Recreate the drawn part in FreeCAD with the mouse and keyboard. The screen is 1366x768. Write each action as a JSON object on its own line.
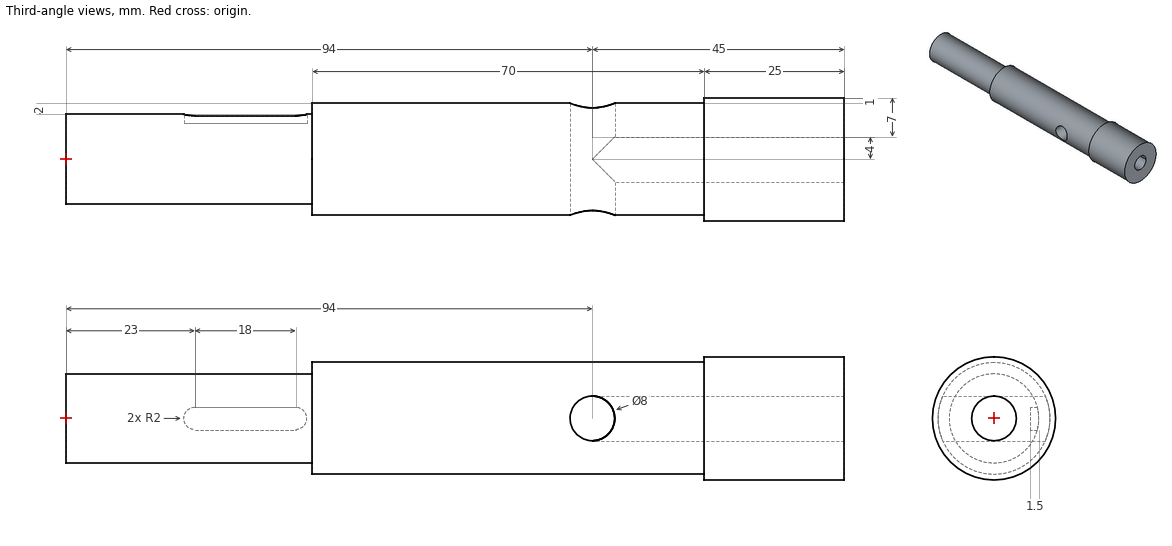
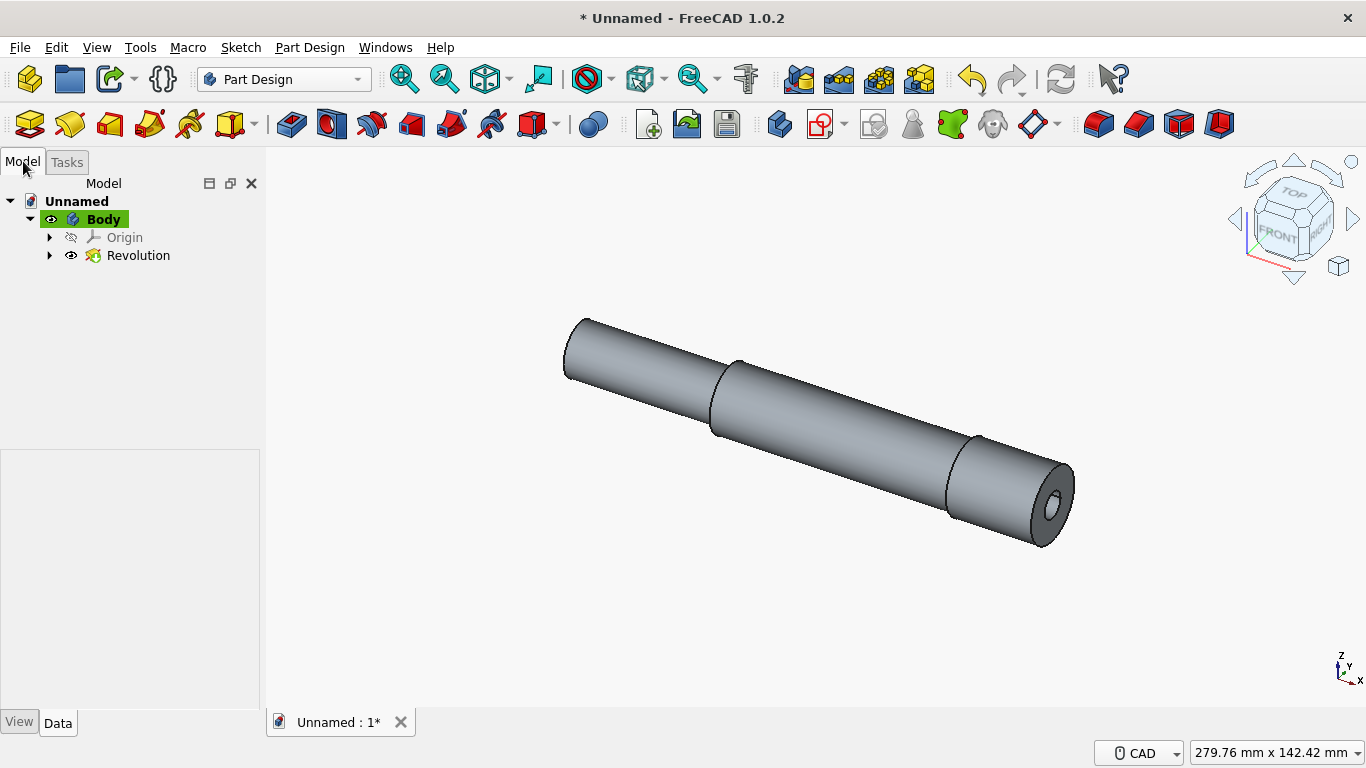
{"action": "left_click", "coordinate": [50, 237]}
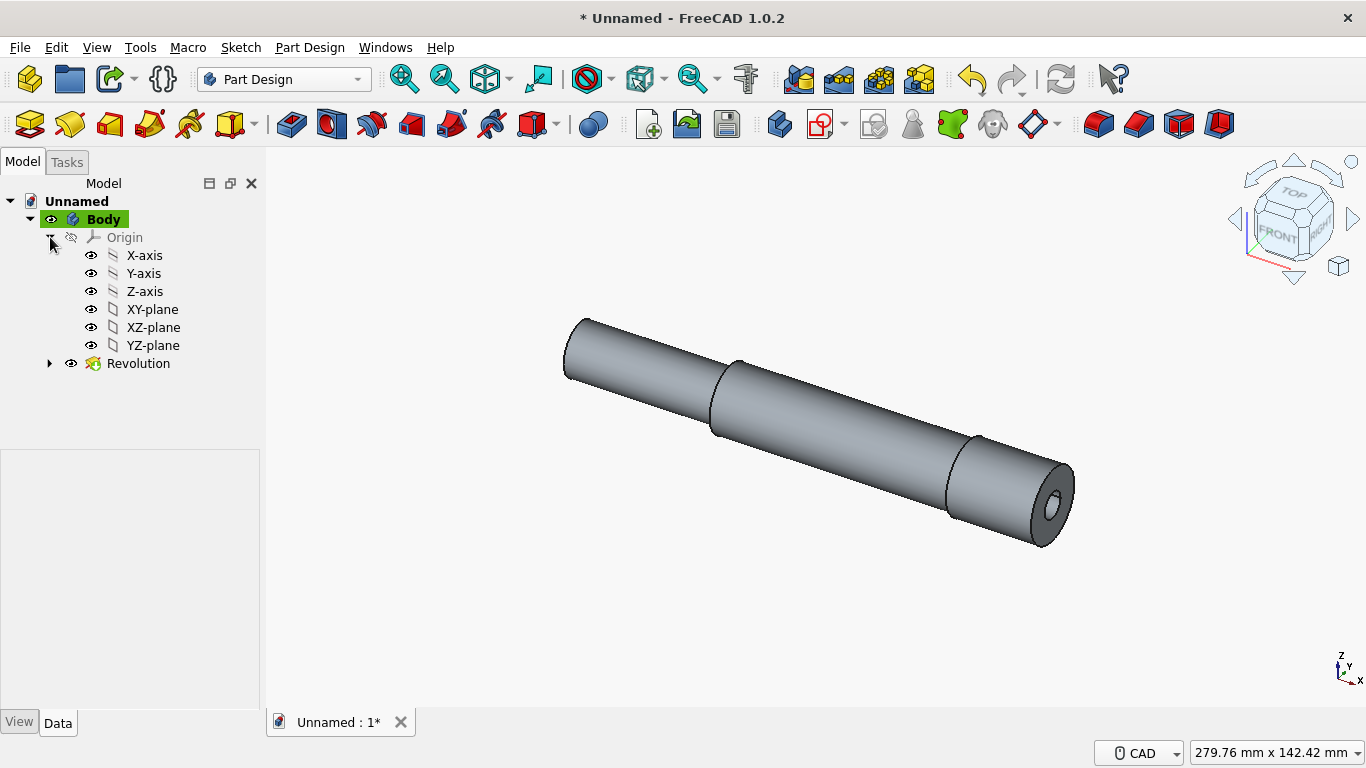
{"action": "left_click", "coordinate": [136, 327]}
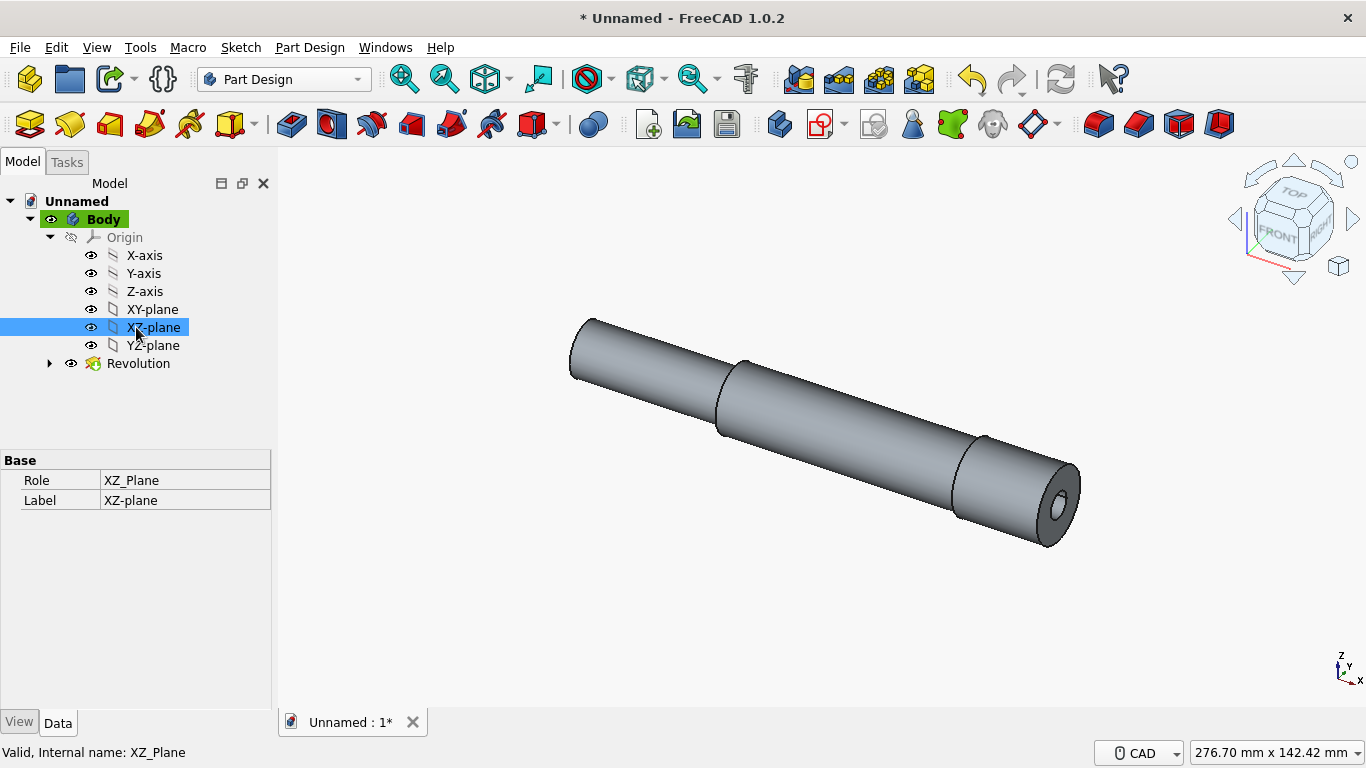
{"action": "left_click", "coordinate": [1034, 124]}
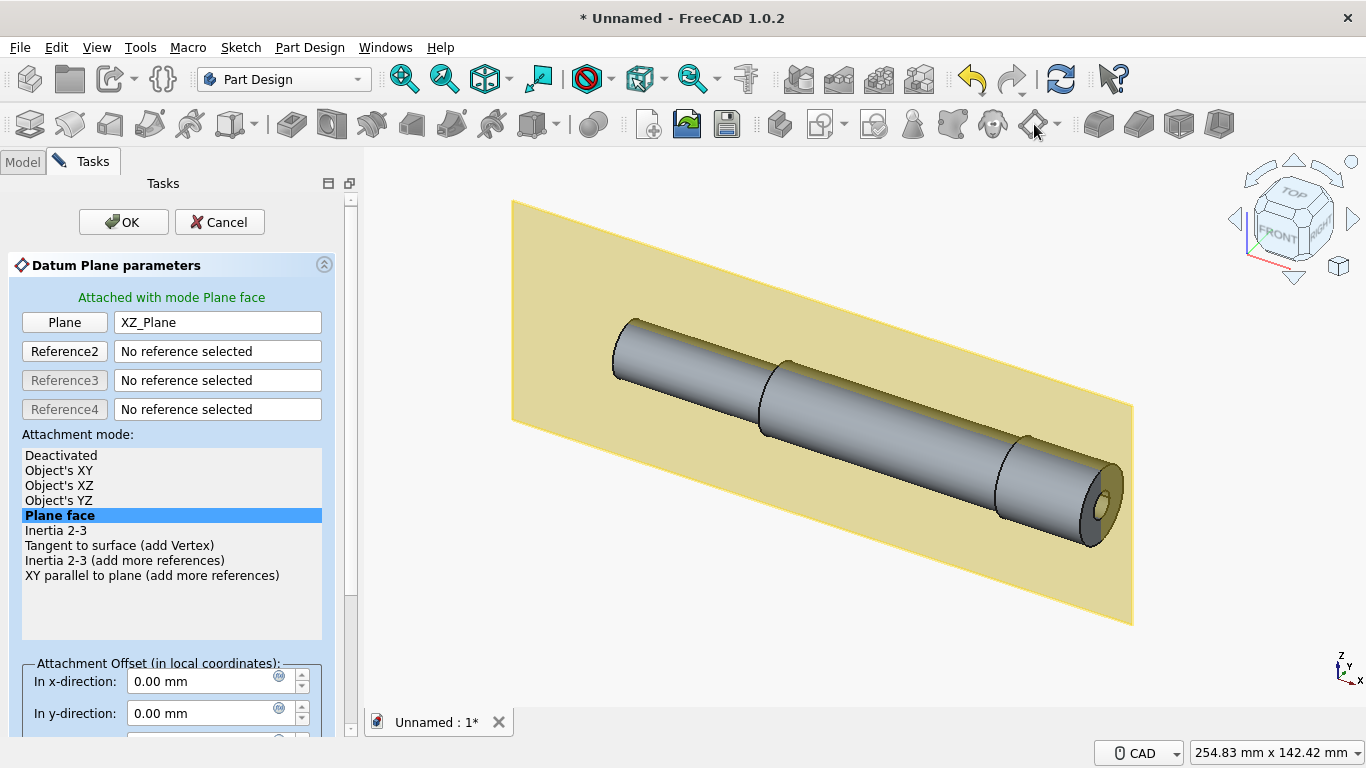
{"action": "scroll", "coordinate": [351, 464], "scroll_direction": "down", "scroll_amount": 2}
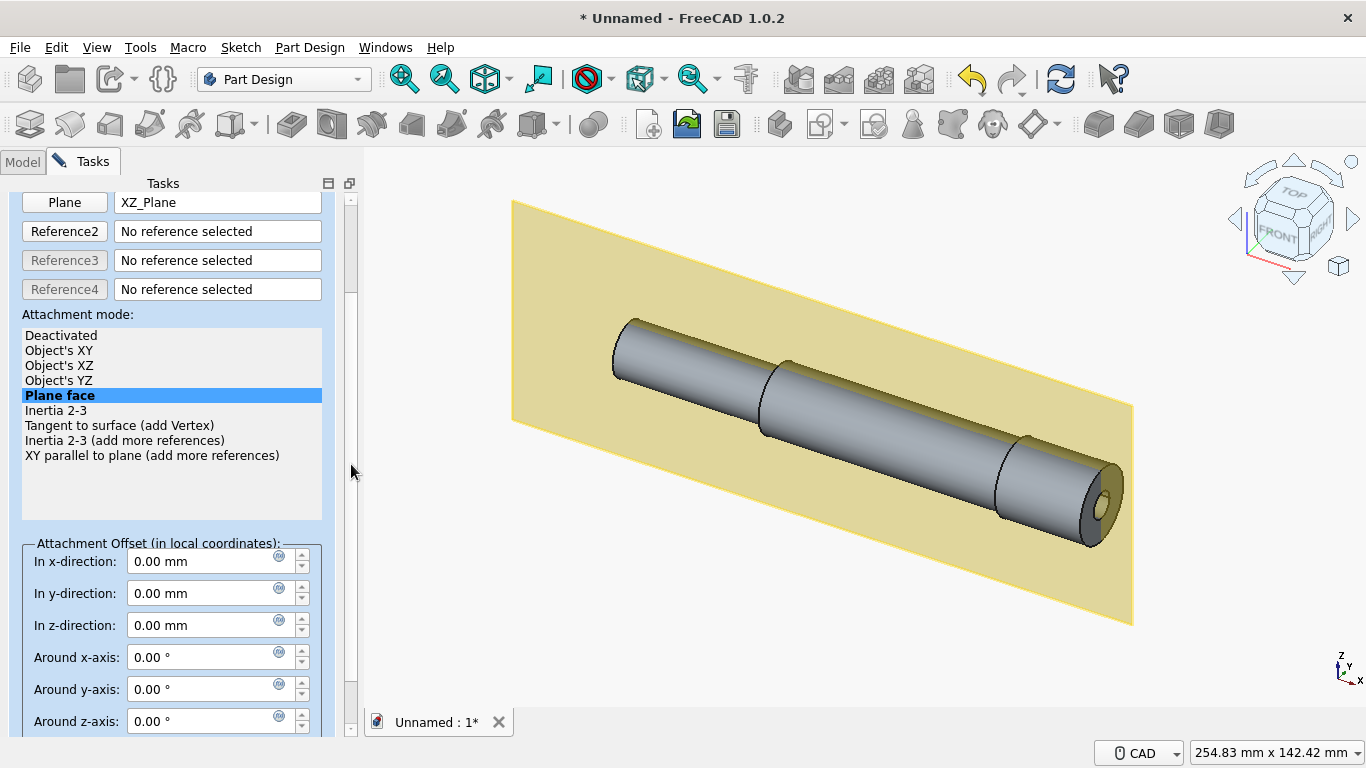
{"action": "triple_click", "coordinate": [210, 625]}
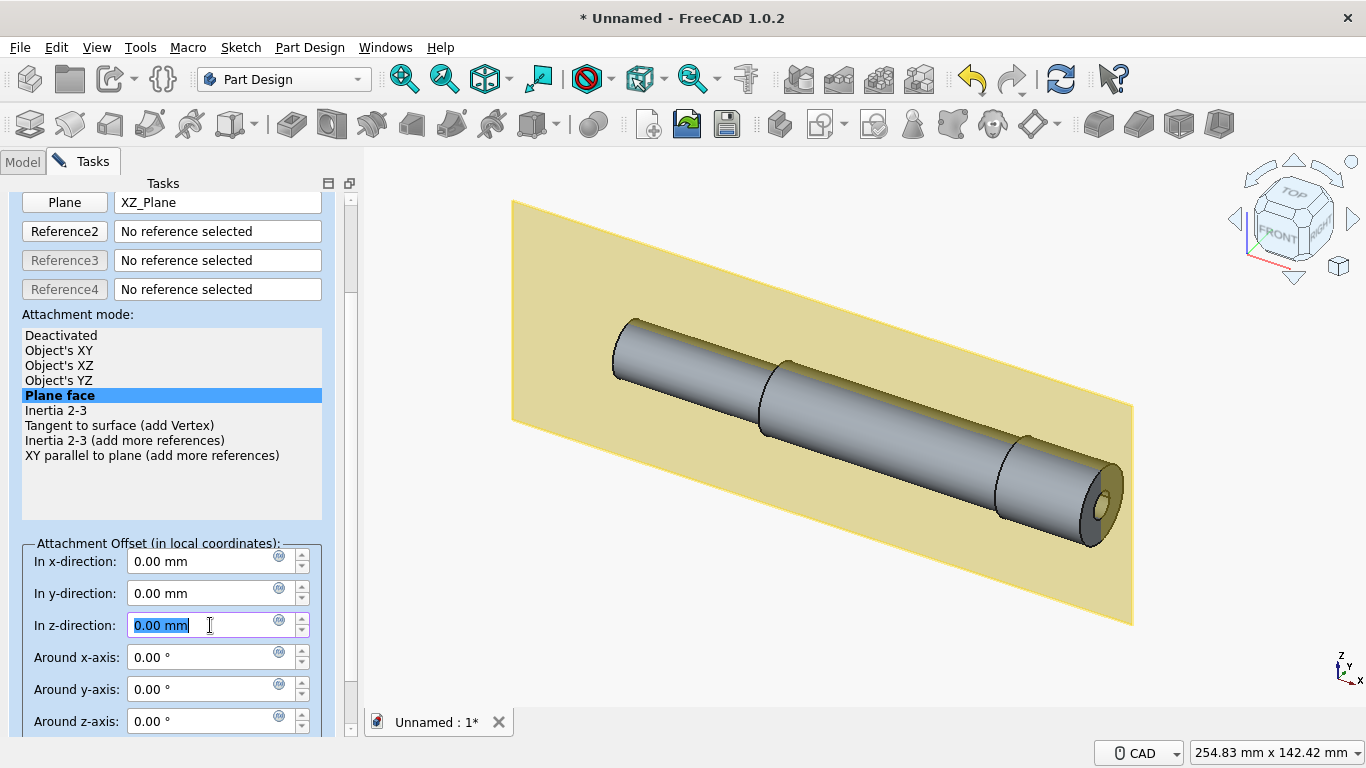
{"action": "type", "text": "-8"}
{"action": "key", "text": "Tab"}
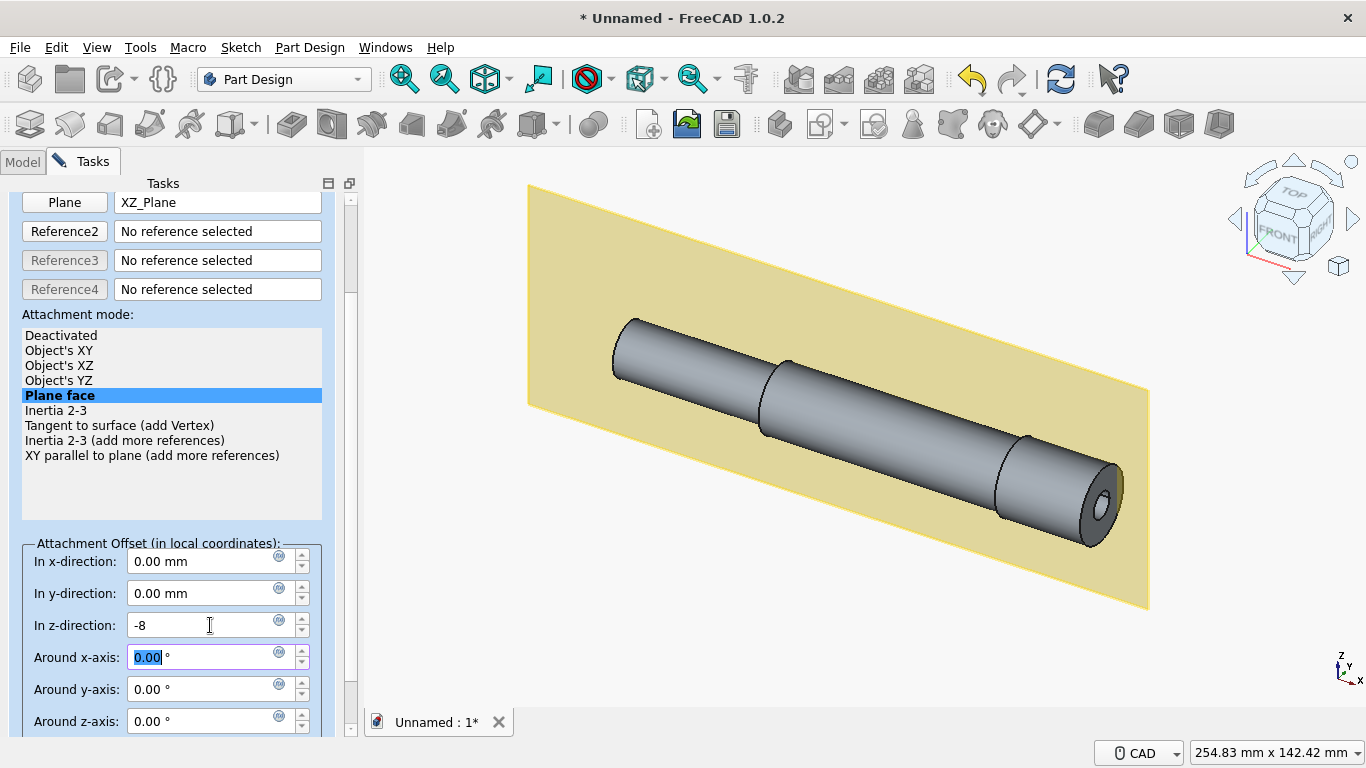
{"action": "scroll", "coordinate": [351, 464], "scroll_direction": "up", "scroll_amount": 3}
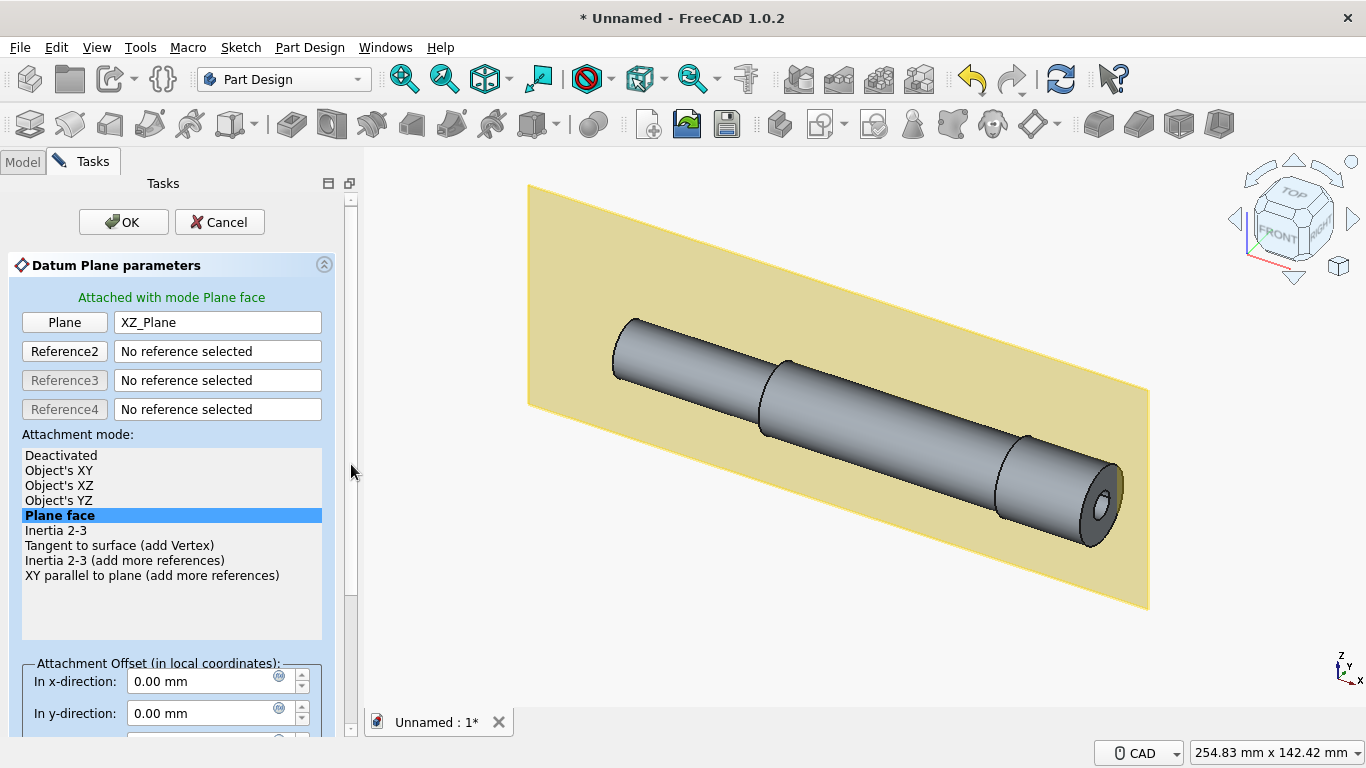
{"action": "left_click", "coordinate": [124, 222]}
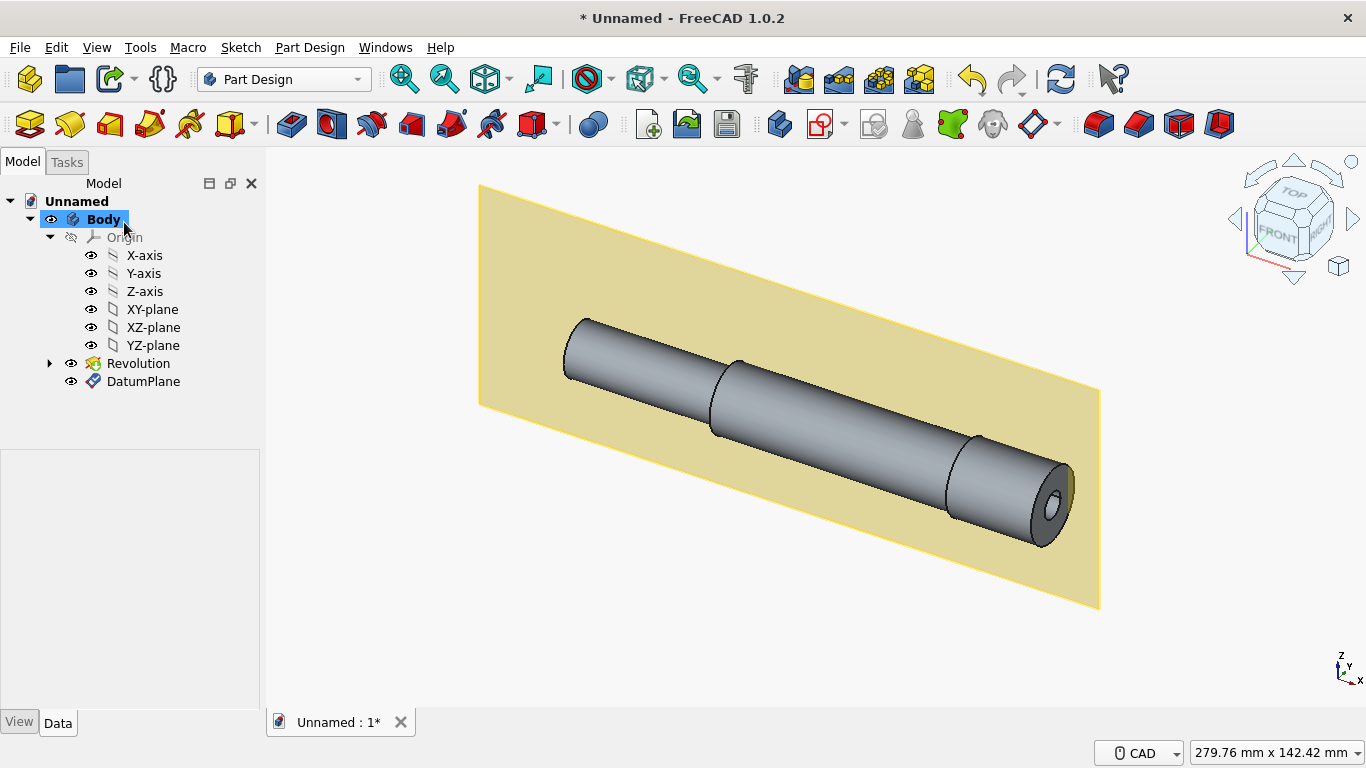
{"action": "left_click", "coordinate": [116, 381]}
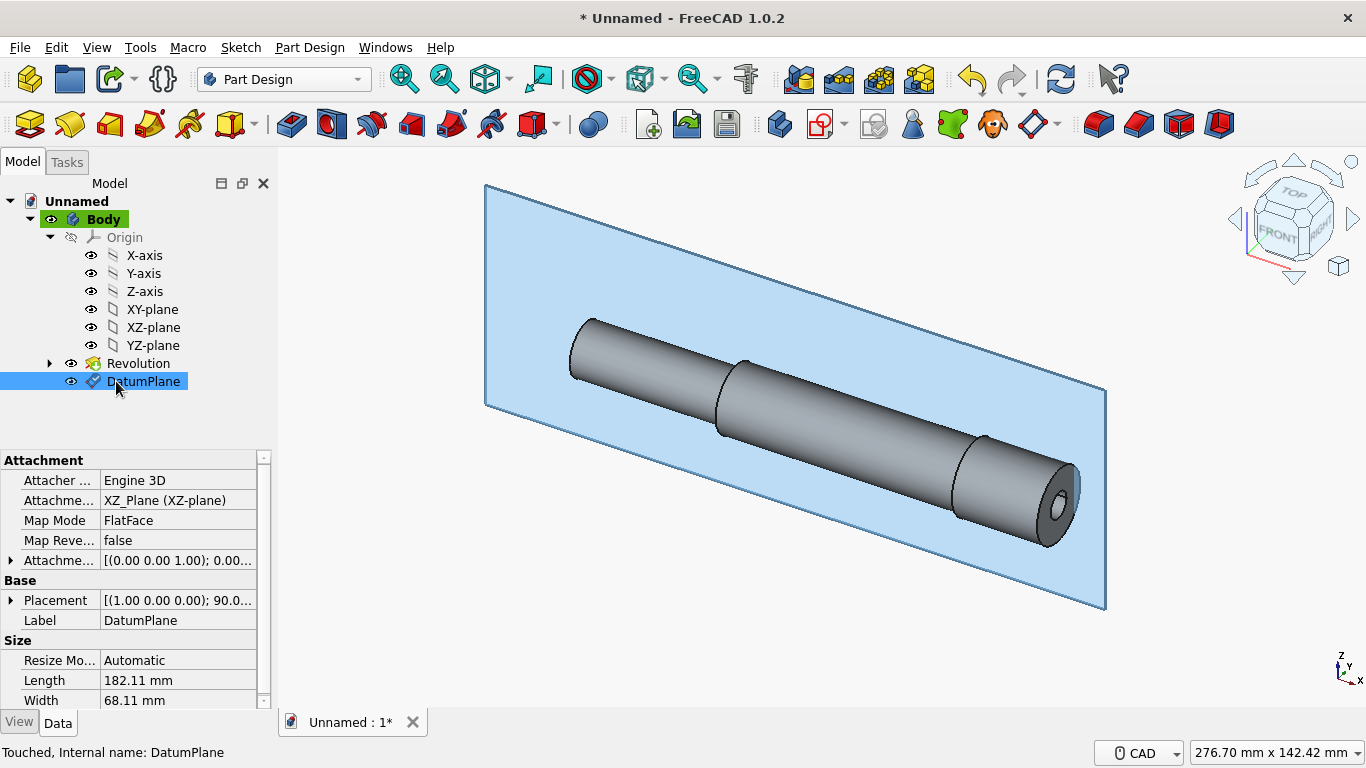
{"action": "left_click", "coordinate": [820, 124]}